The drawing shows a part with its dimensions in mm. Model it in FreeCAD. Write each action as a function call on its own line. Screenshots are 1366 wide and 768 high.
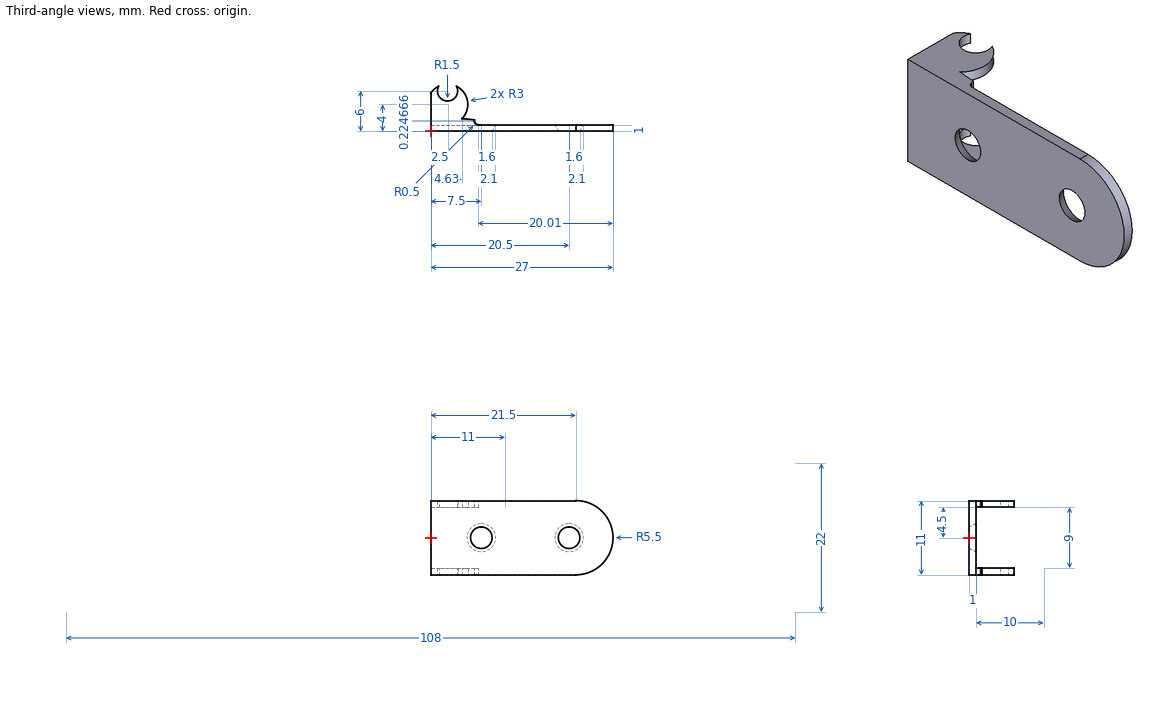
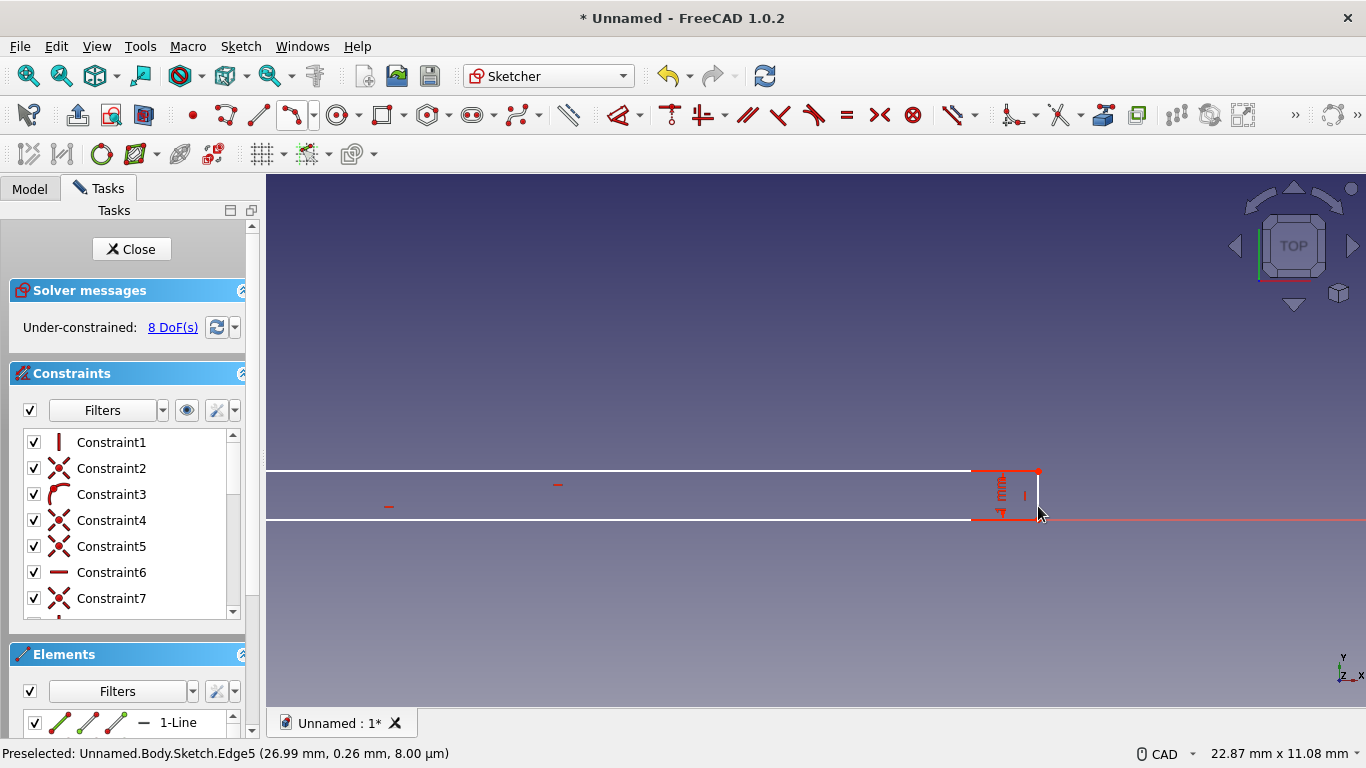
click(649, 520)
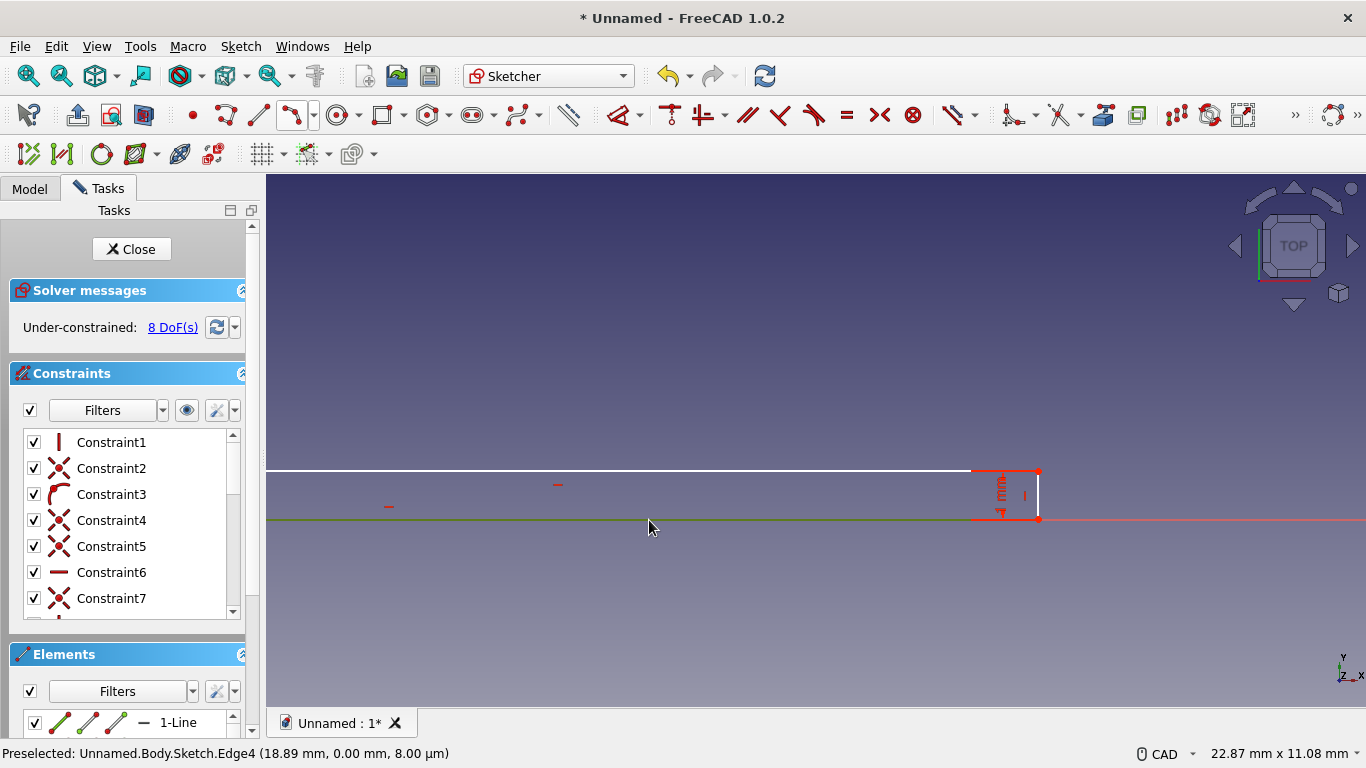
click(640, 116)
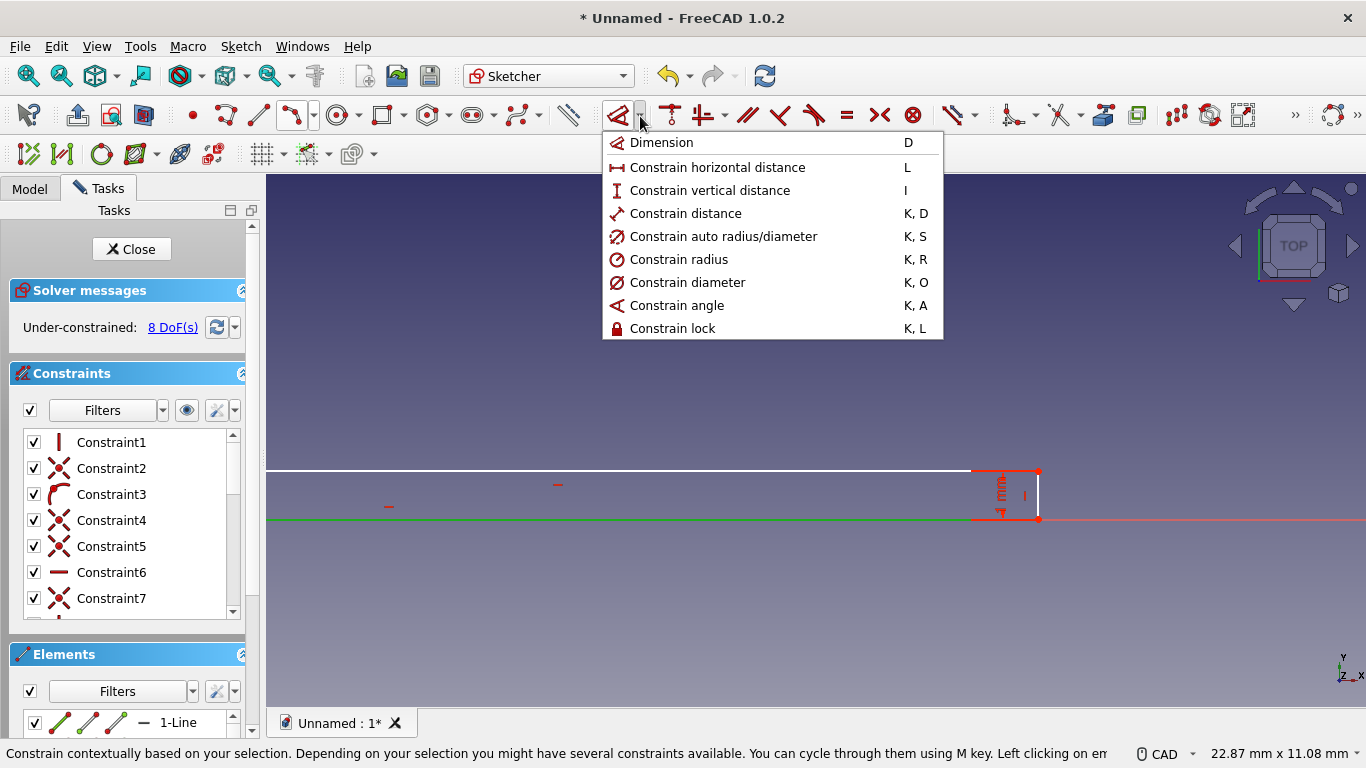
click(773, 168)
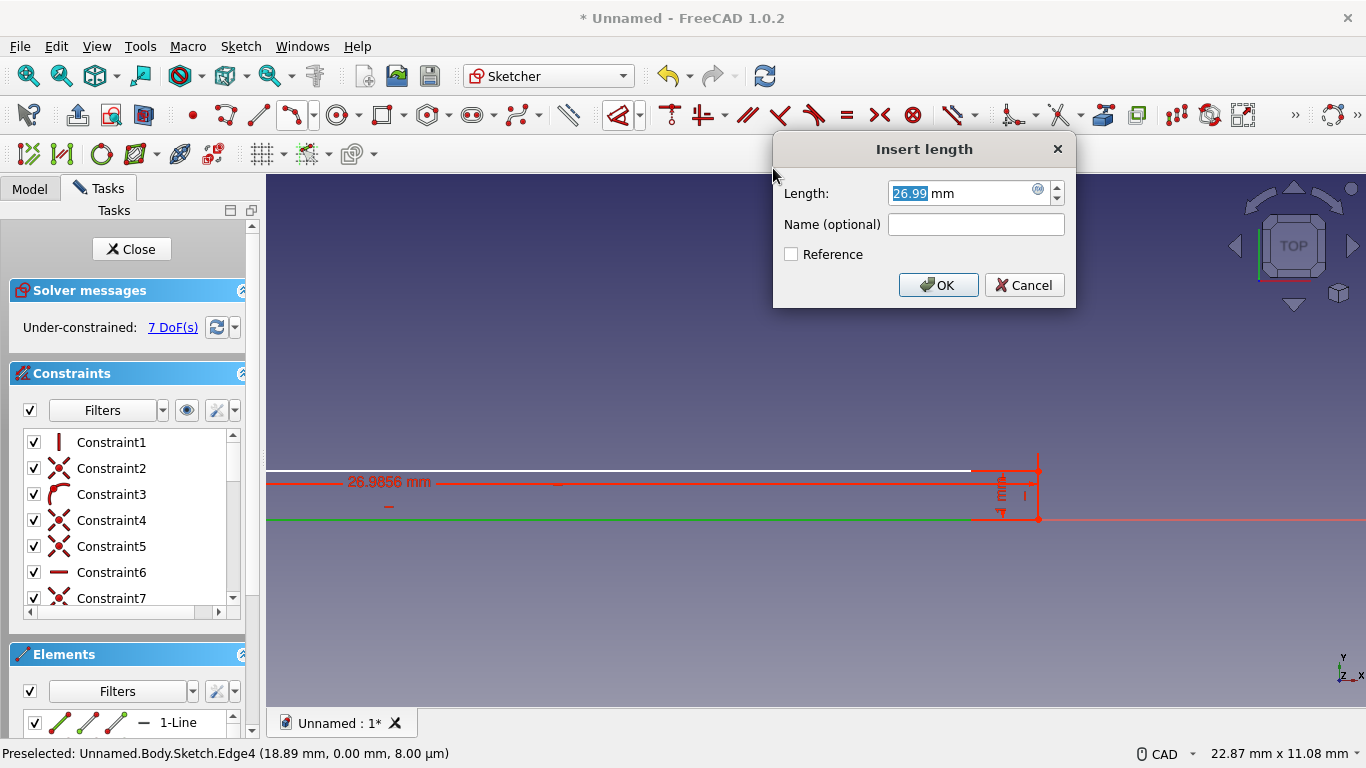
text(27)
key(Return)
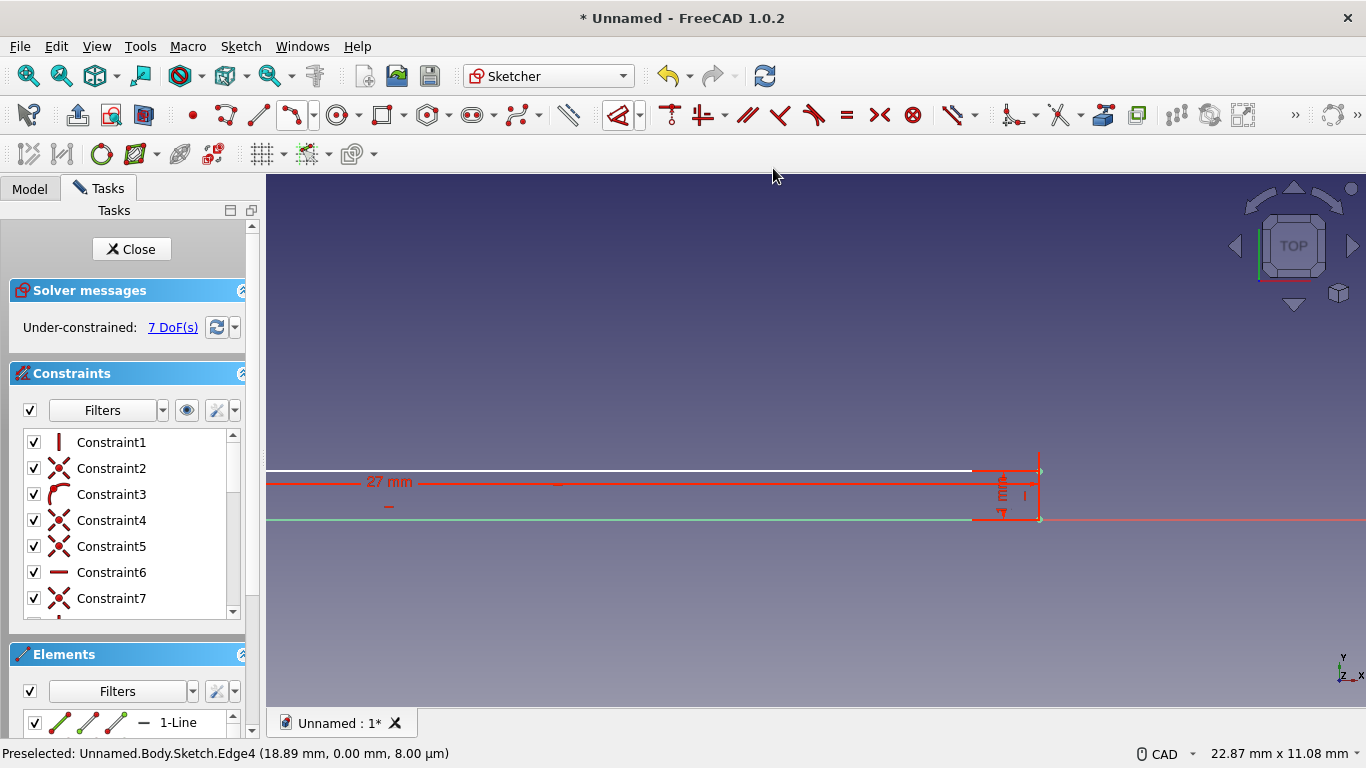
scroll(1039, 507, down, 4)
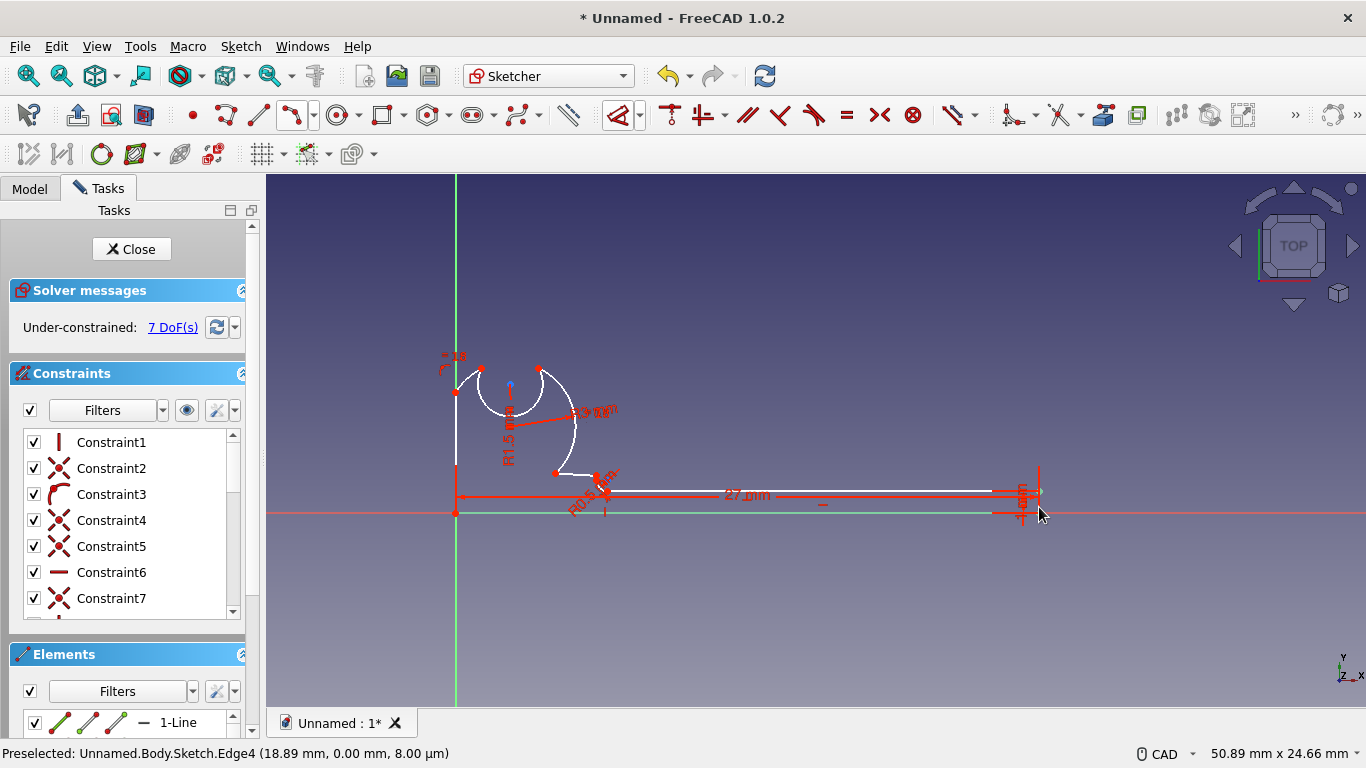
click(511, 427)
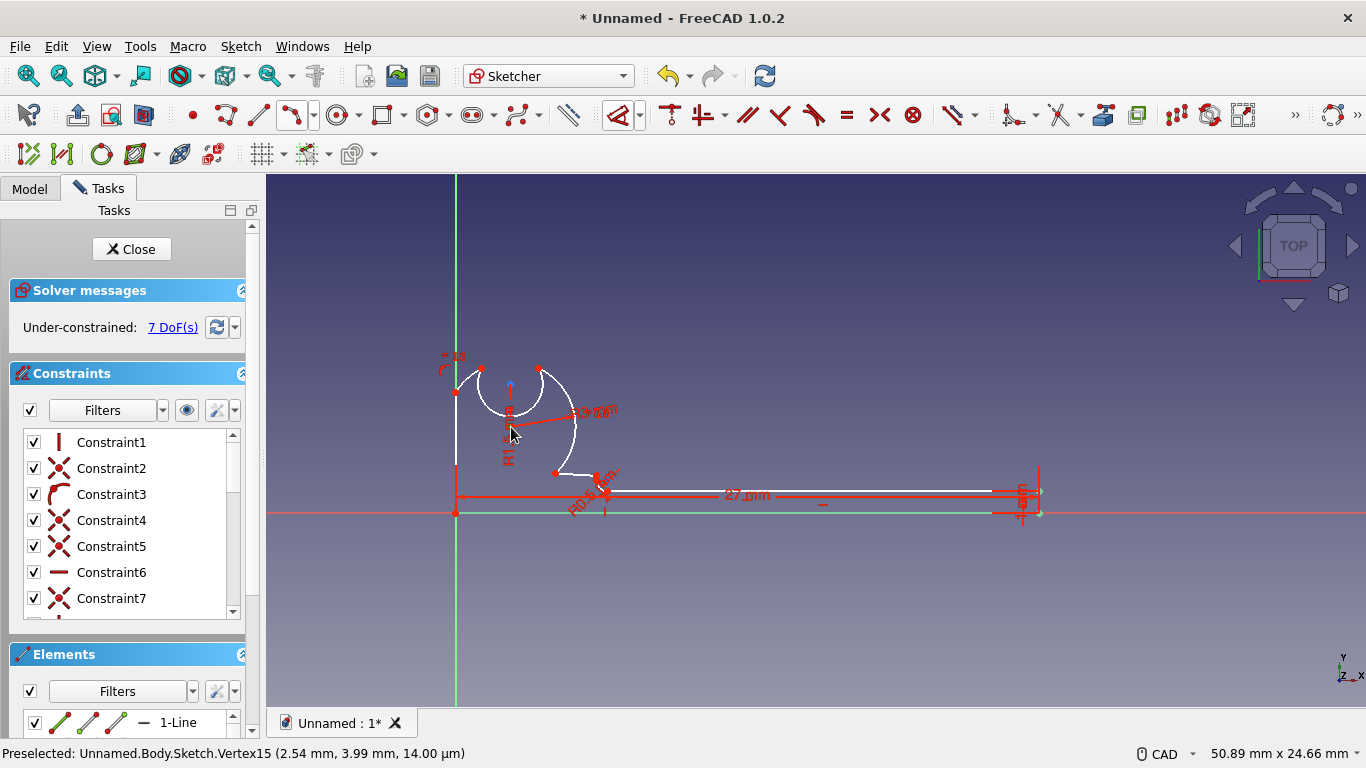
key(i)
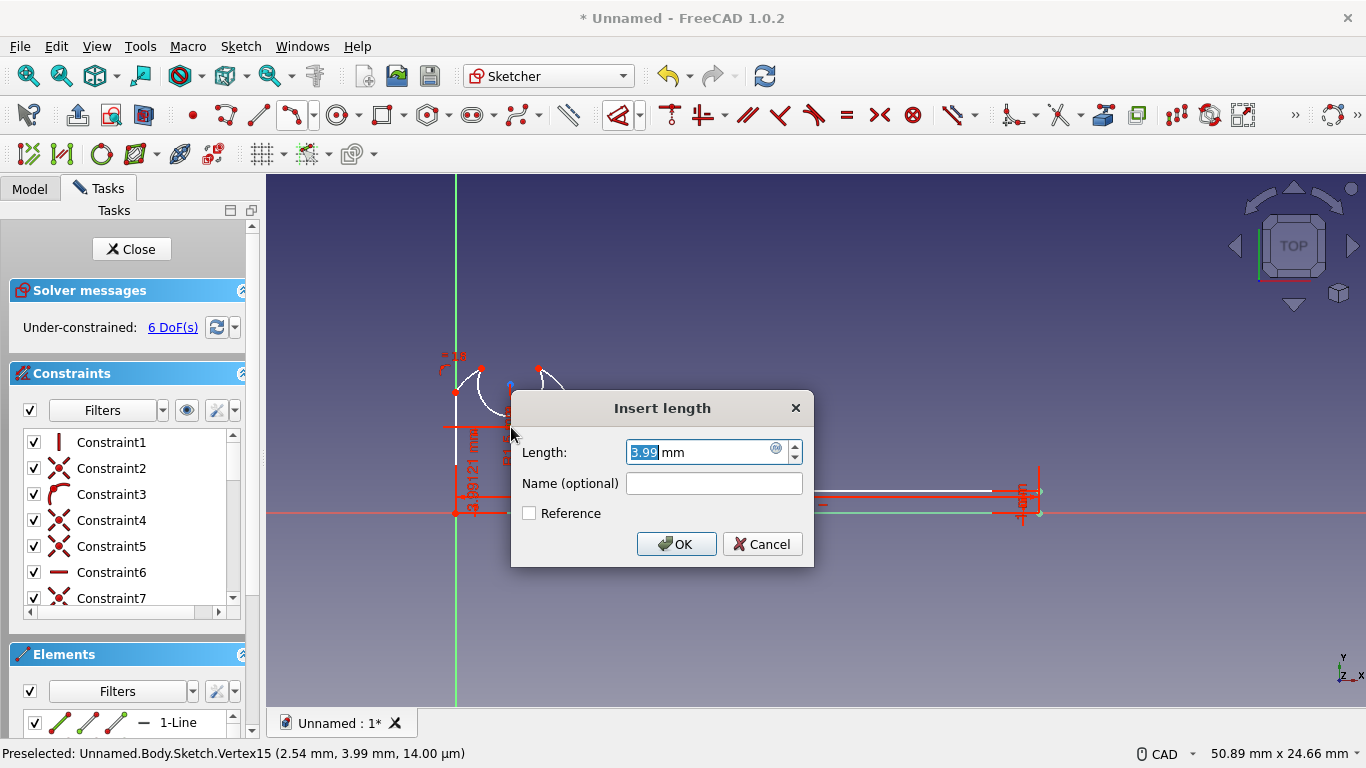
text(4)
key(Return)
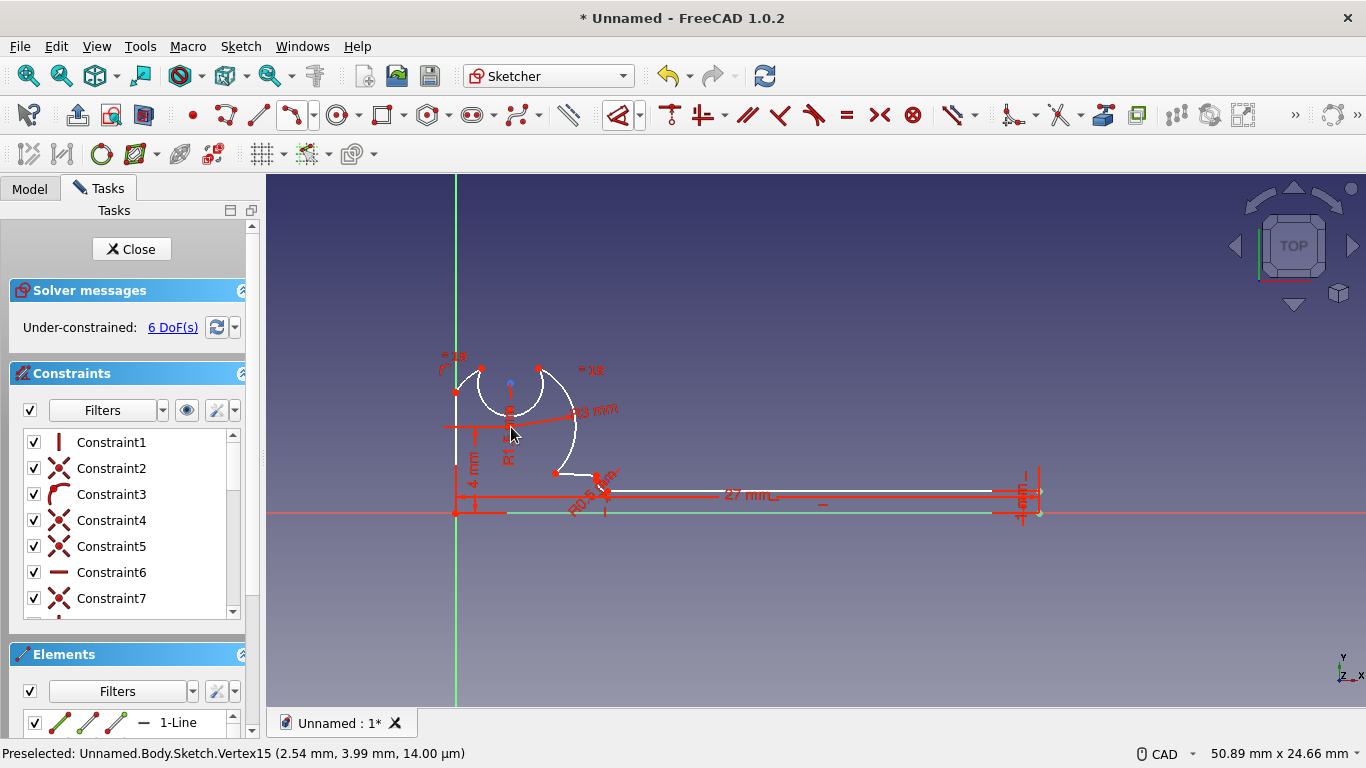
click(510, 384)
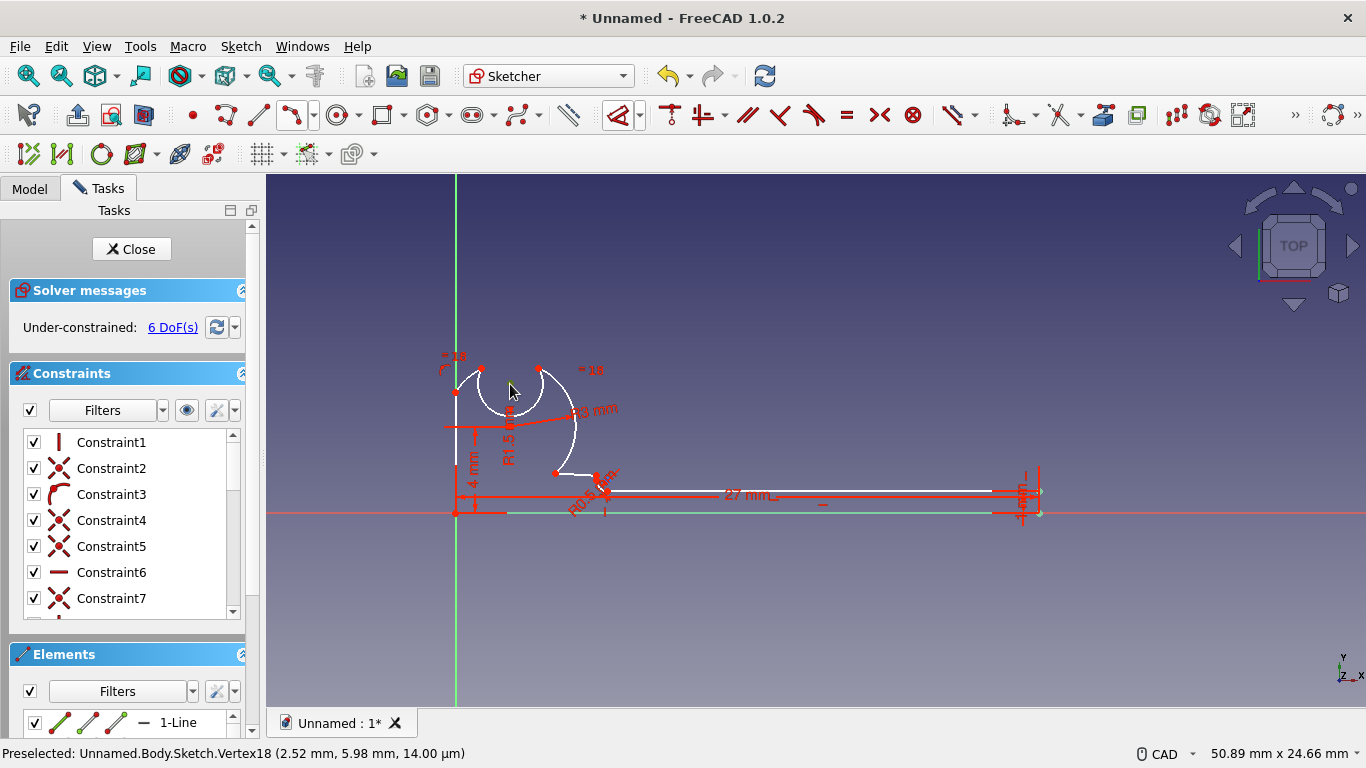
key(i)